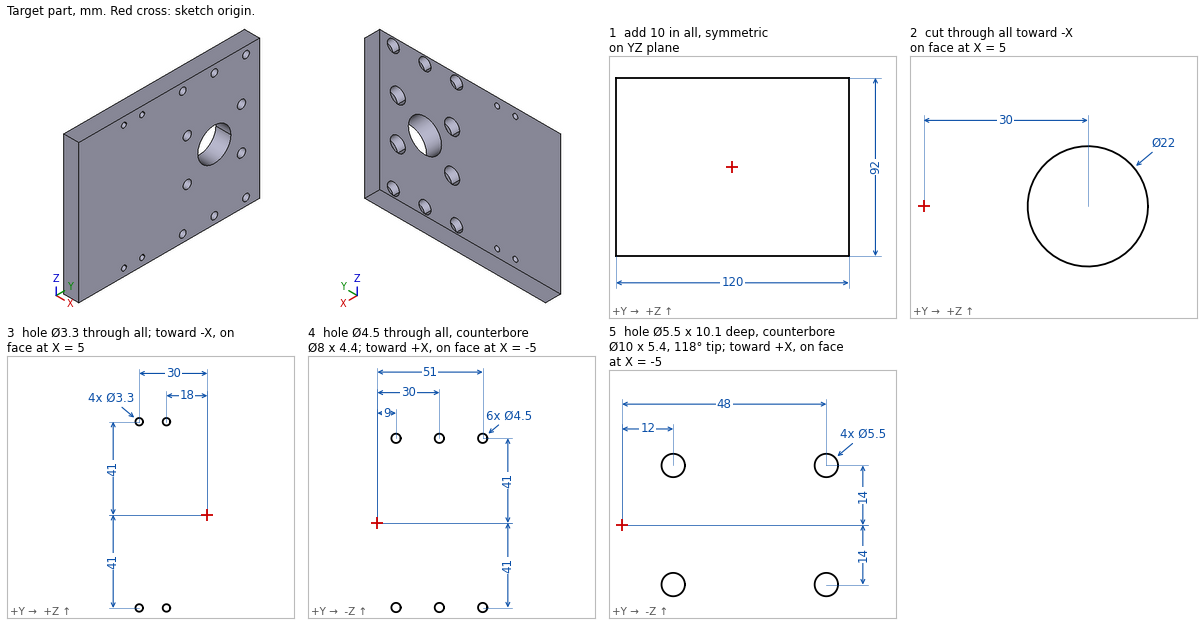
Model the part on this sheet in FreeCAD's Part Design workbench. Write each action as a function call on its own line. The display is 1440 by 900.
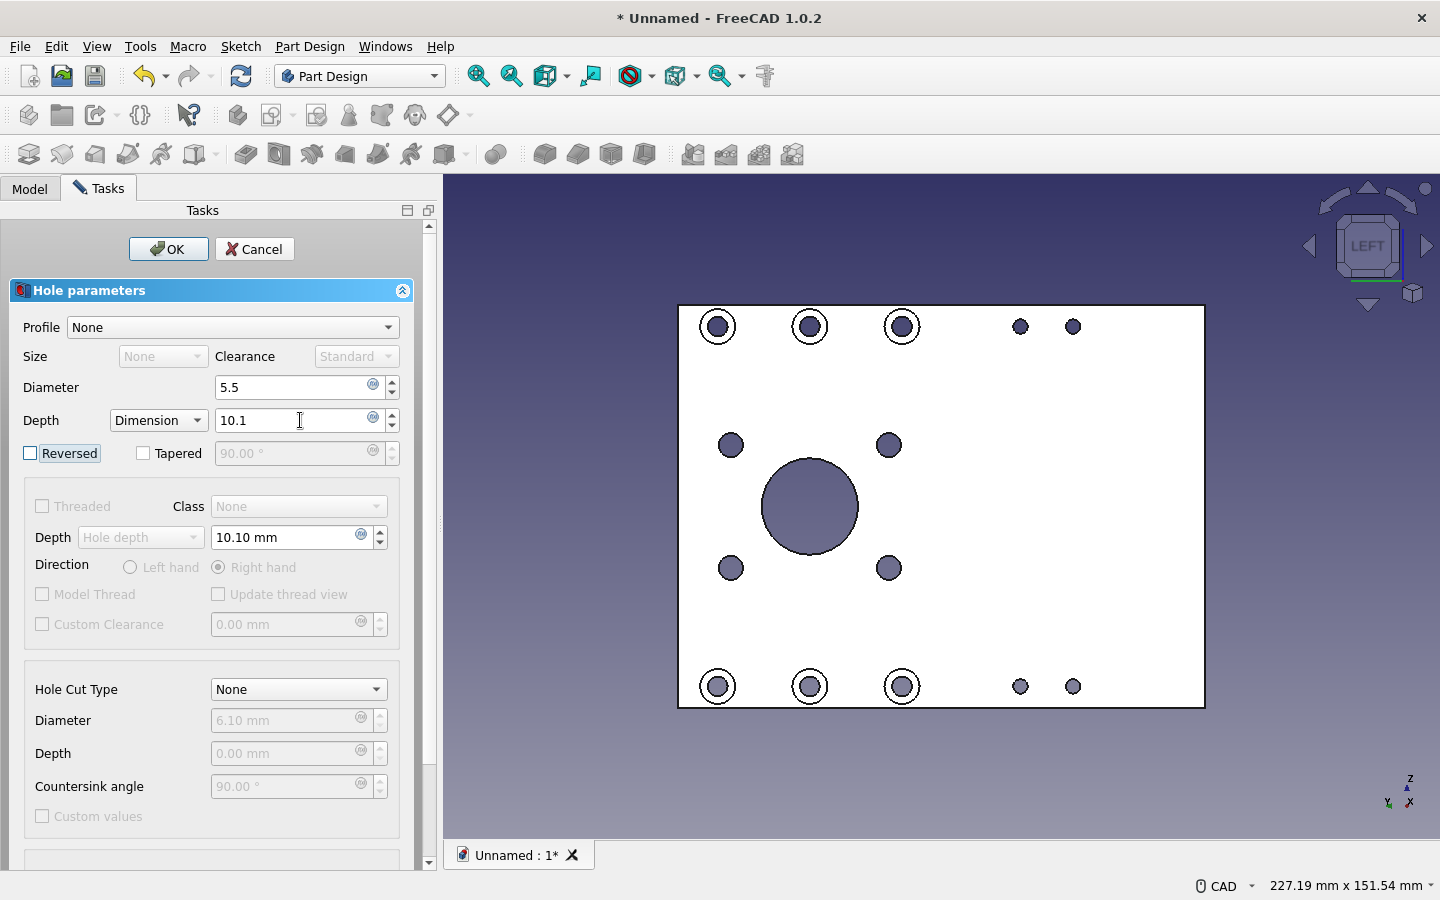
click(300, 690)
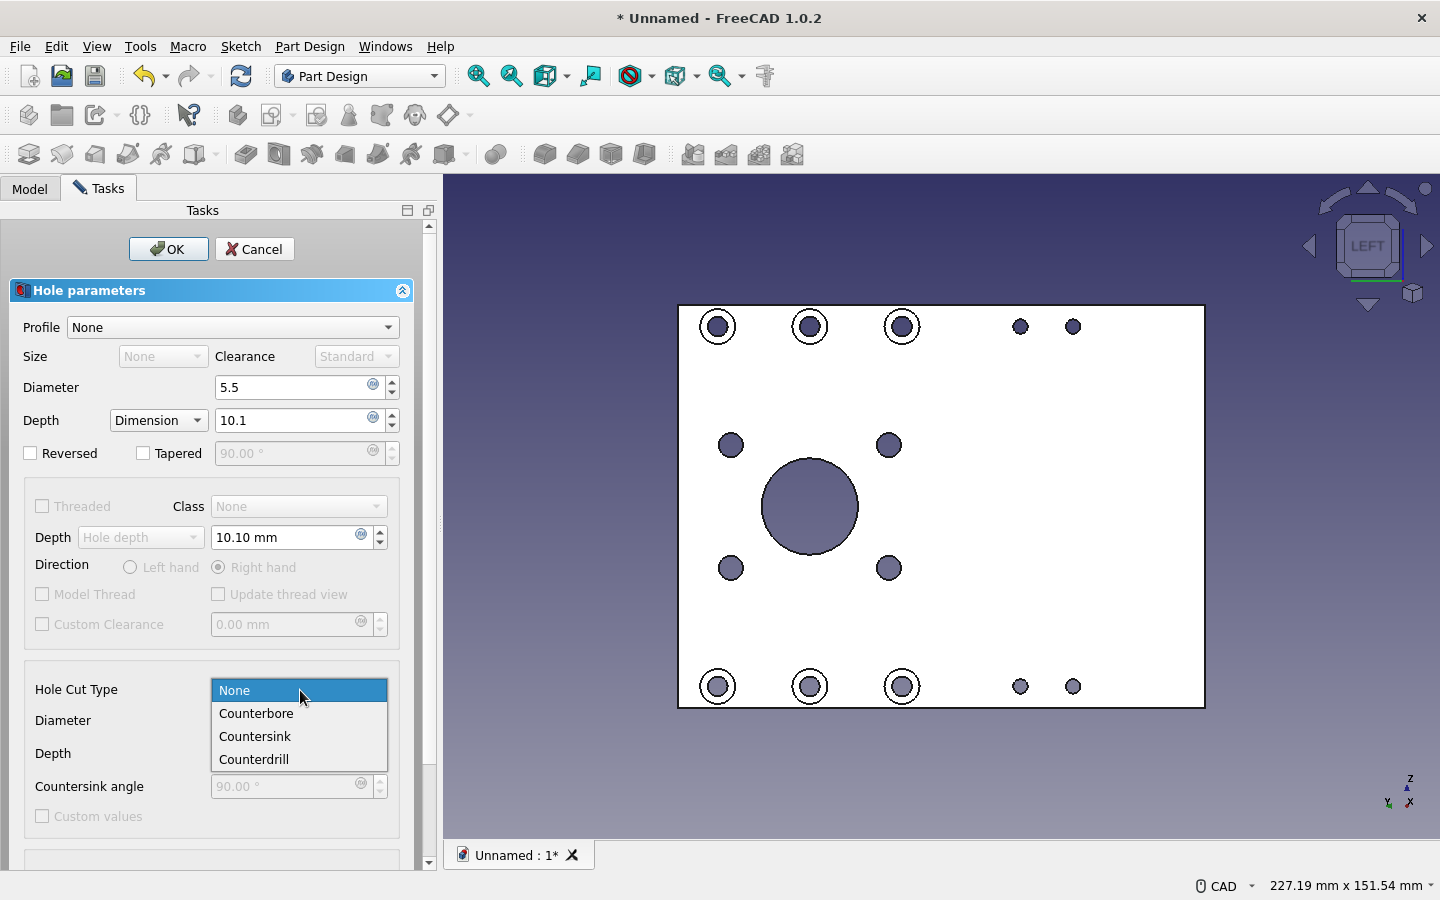
click(298, 714)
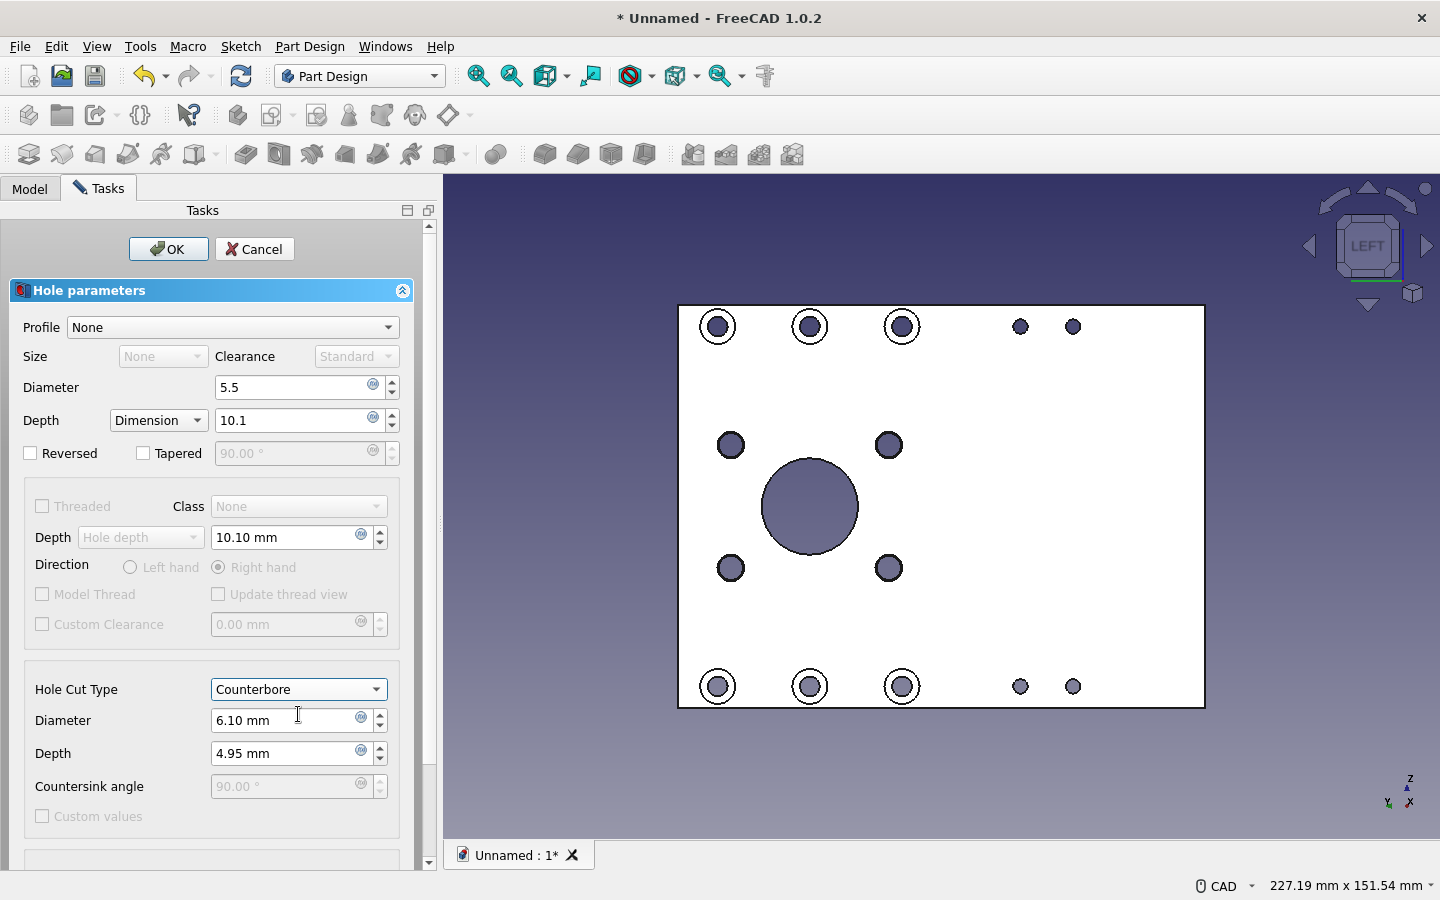
triple_click(292, 720)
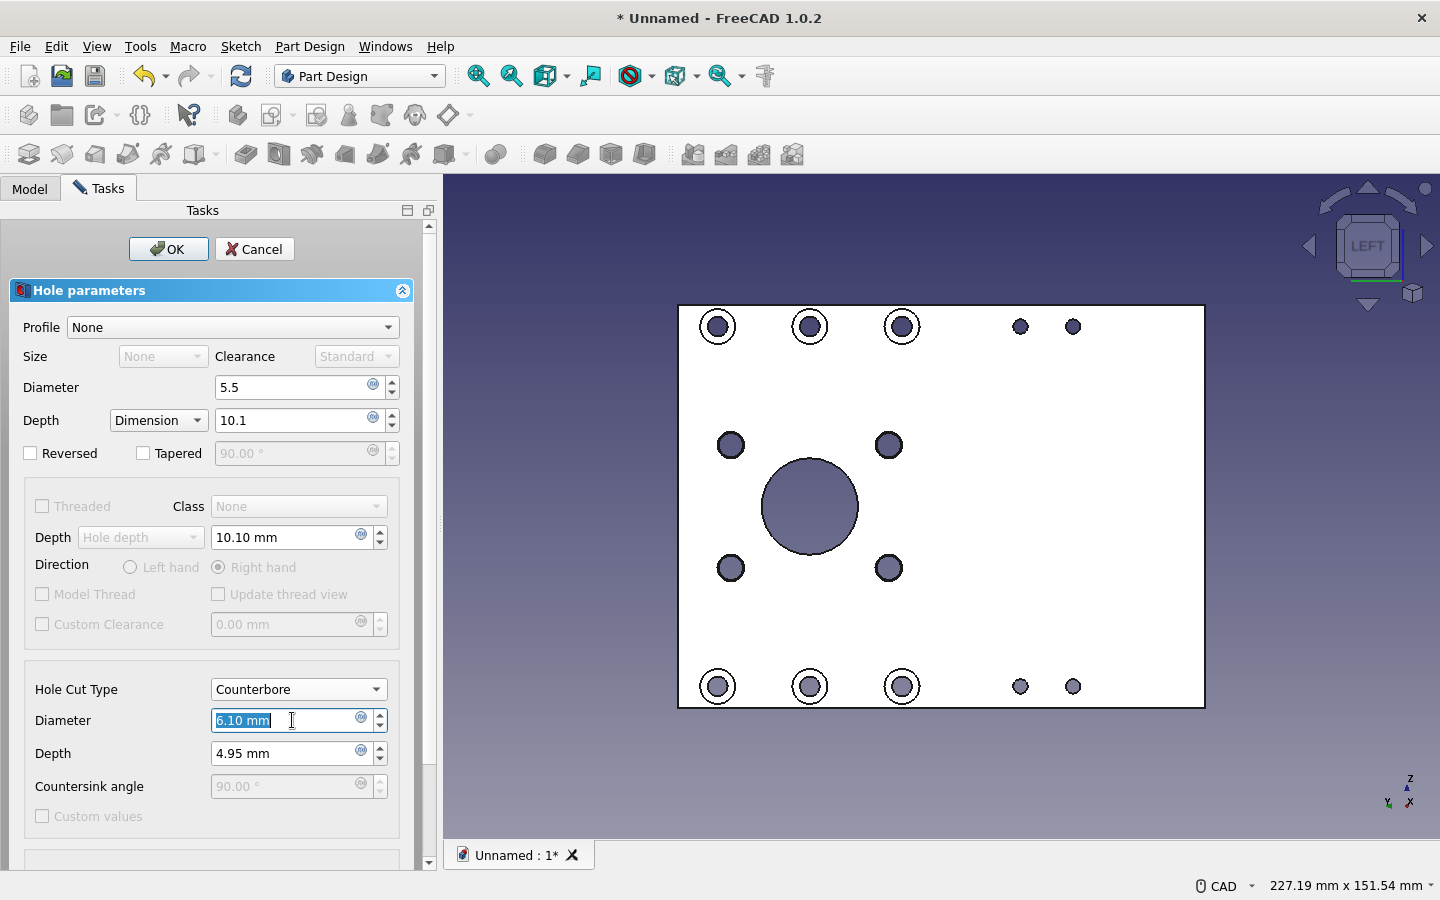
text(10)
key(Tab)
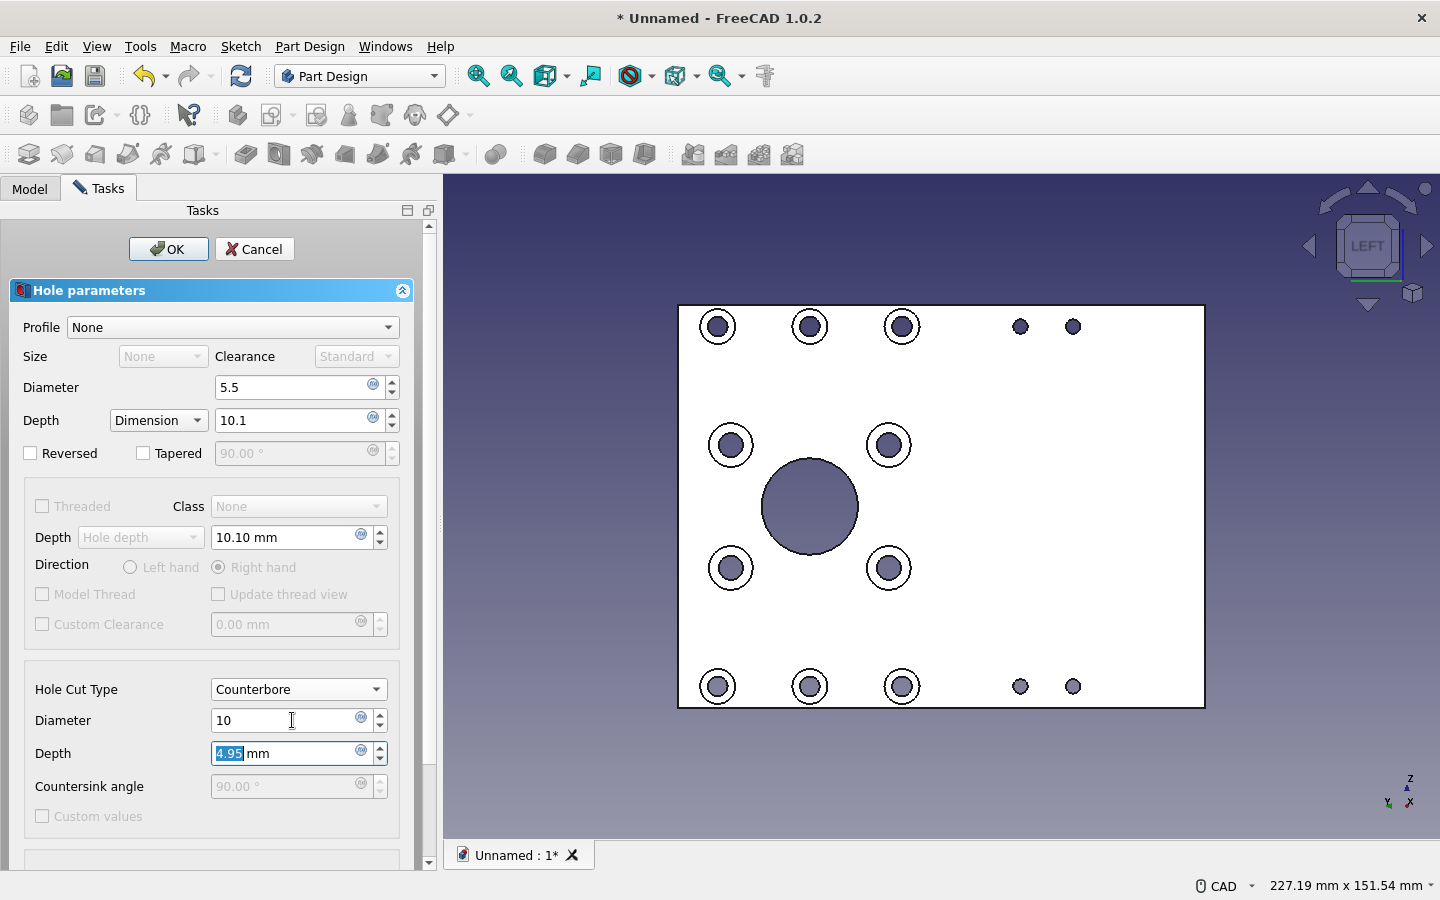
text(5.4)
key(Tab)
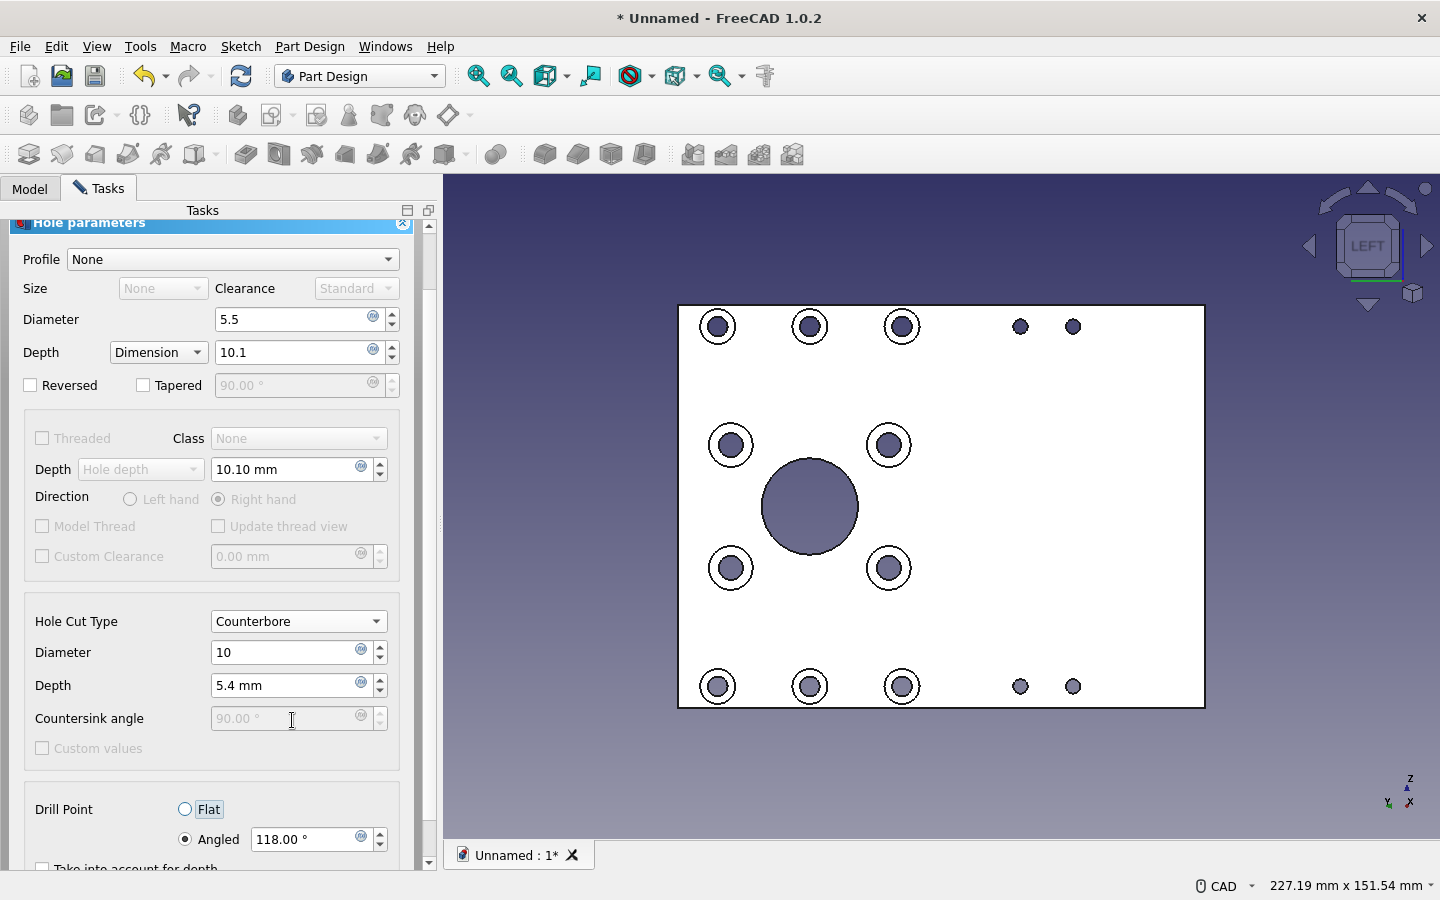
scroll(429, 545, up, 2)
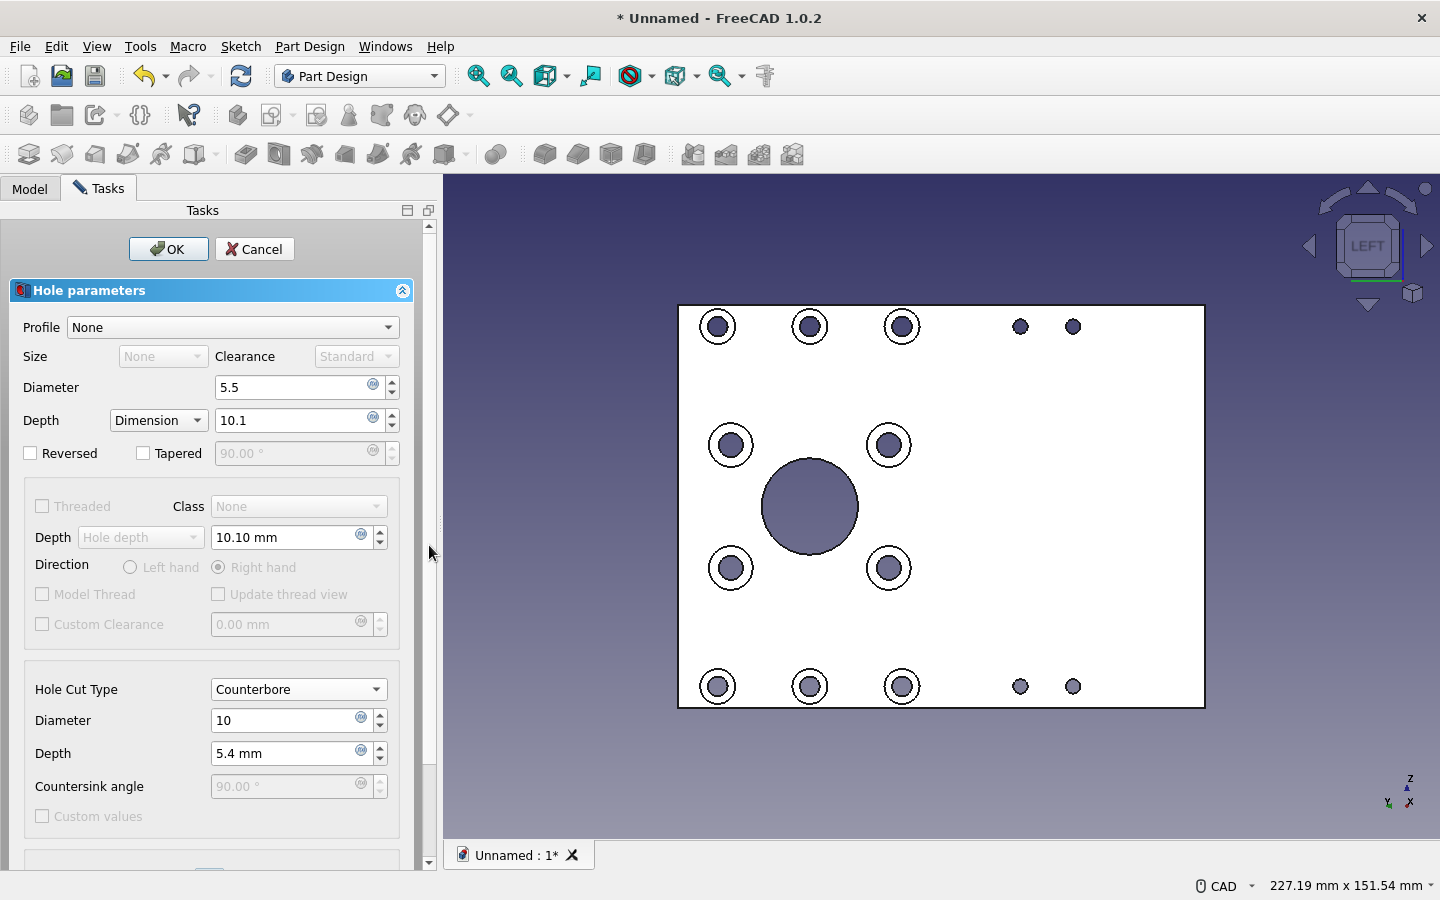
click(169, 249)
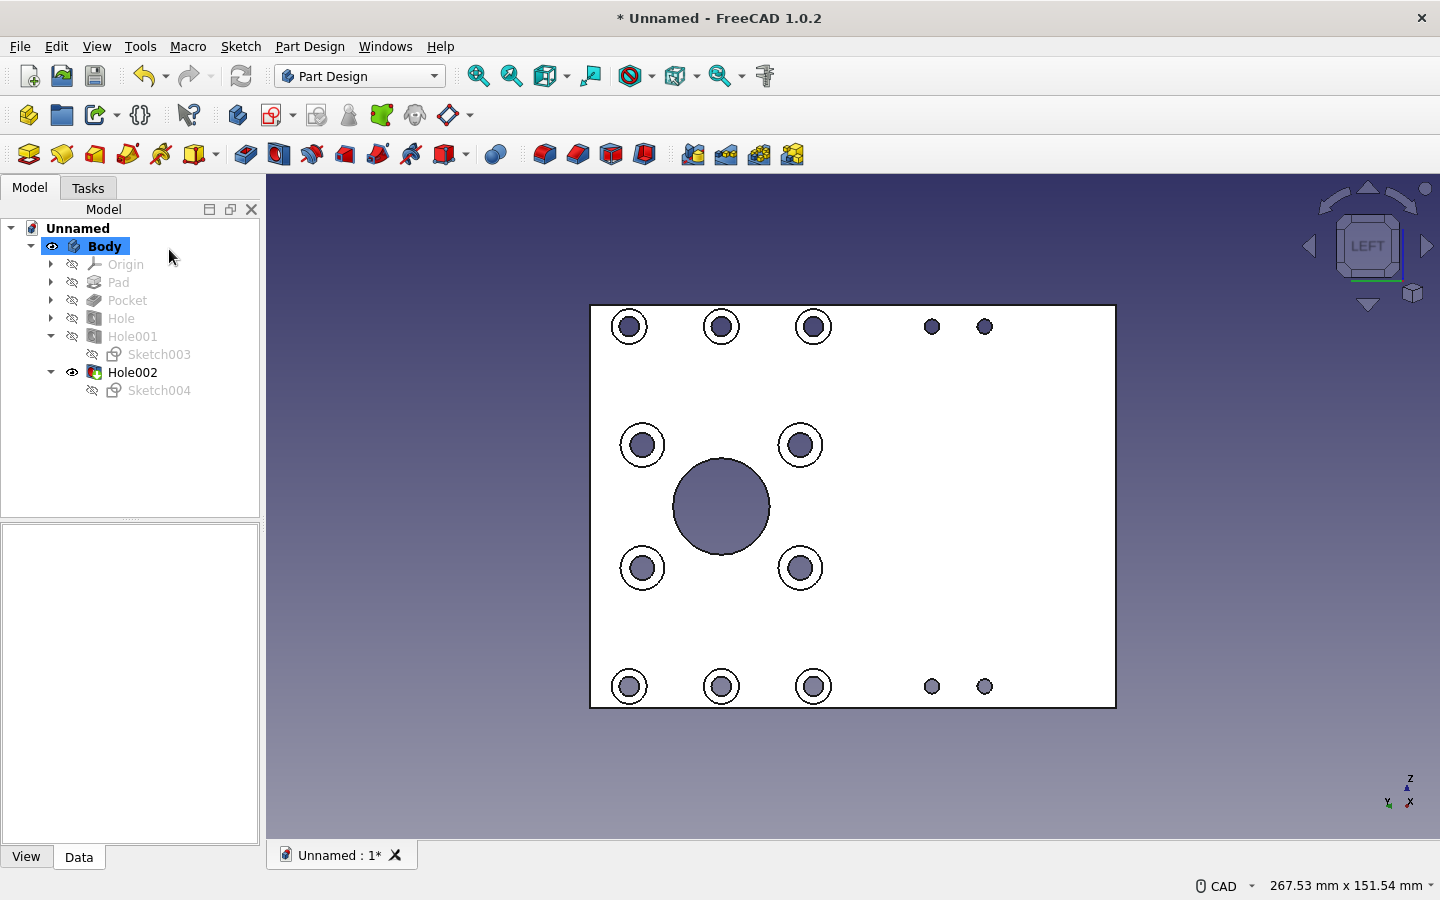
key(0)